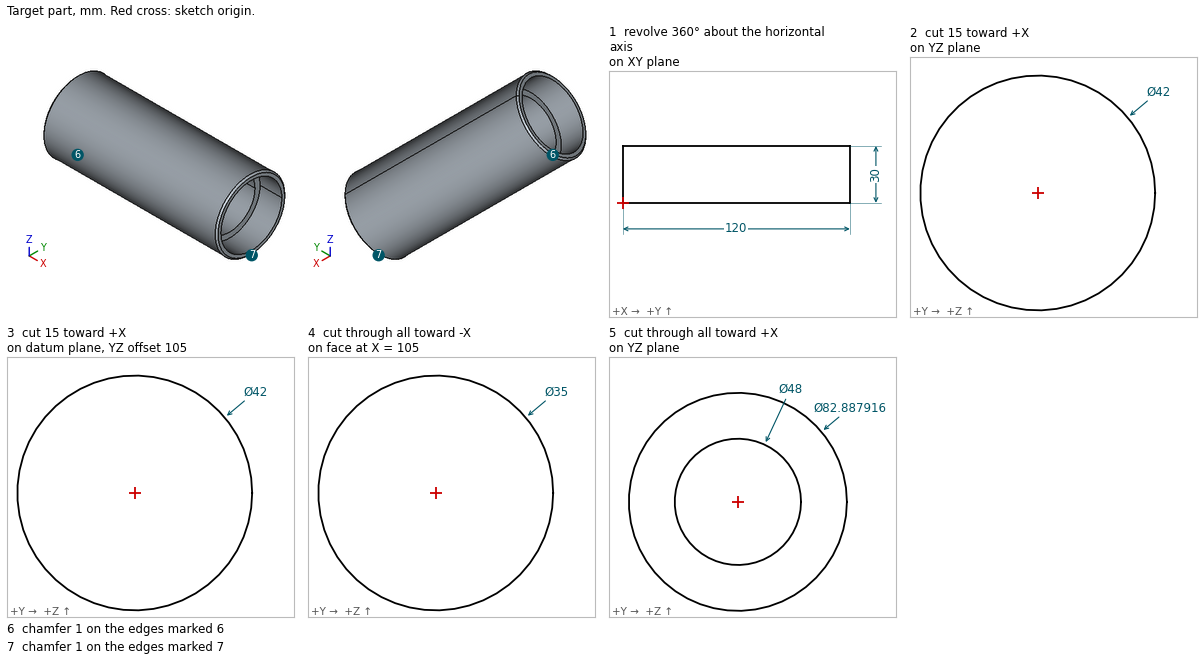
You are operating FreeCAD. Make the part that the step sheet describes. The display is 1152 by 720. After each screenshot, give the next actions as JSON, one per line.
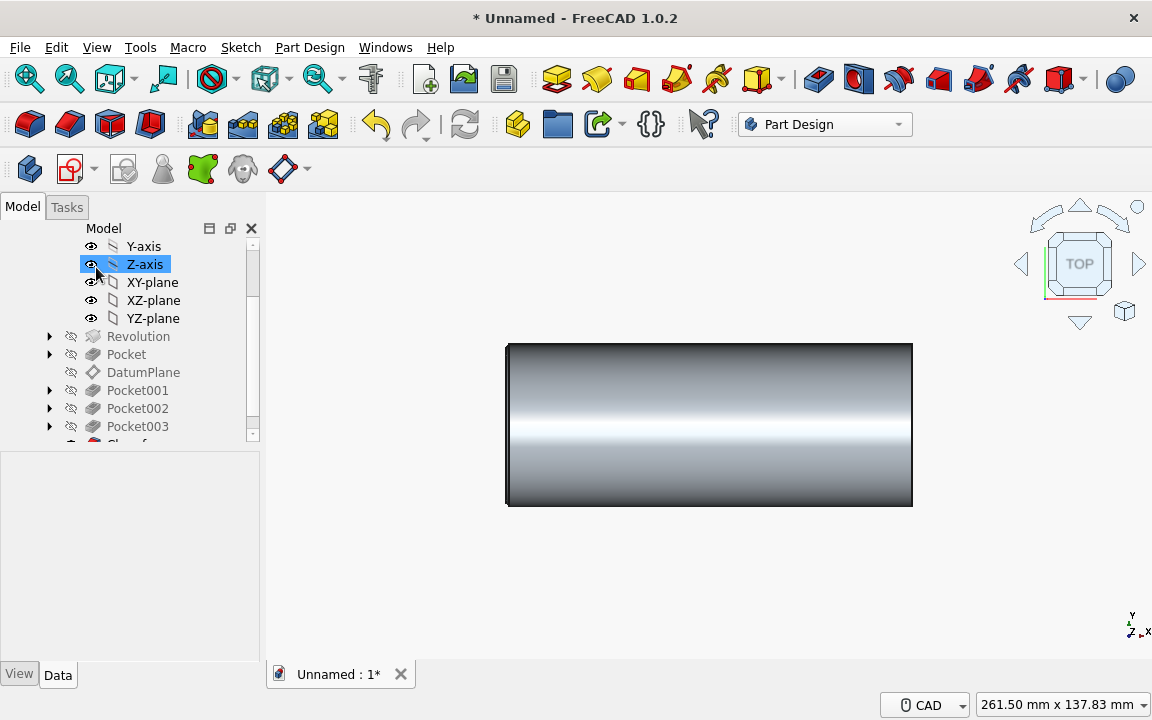
{"action": "left_click", "coordinate": [912, 490]}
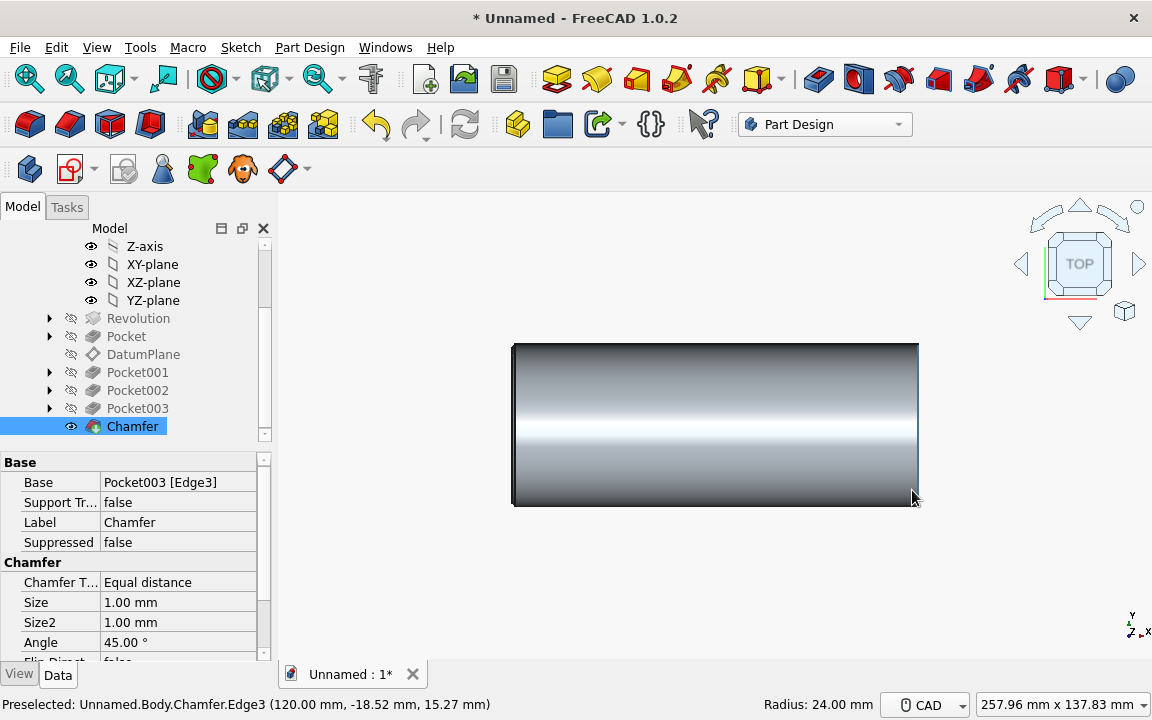
{"action": "left_click", "coordinate": [70, 124]}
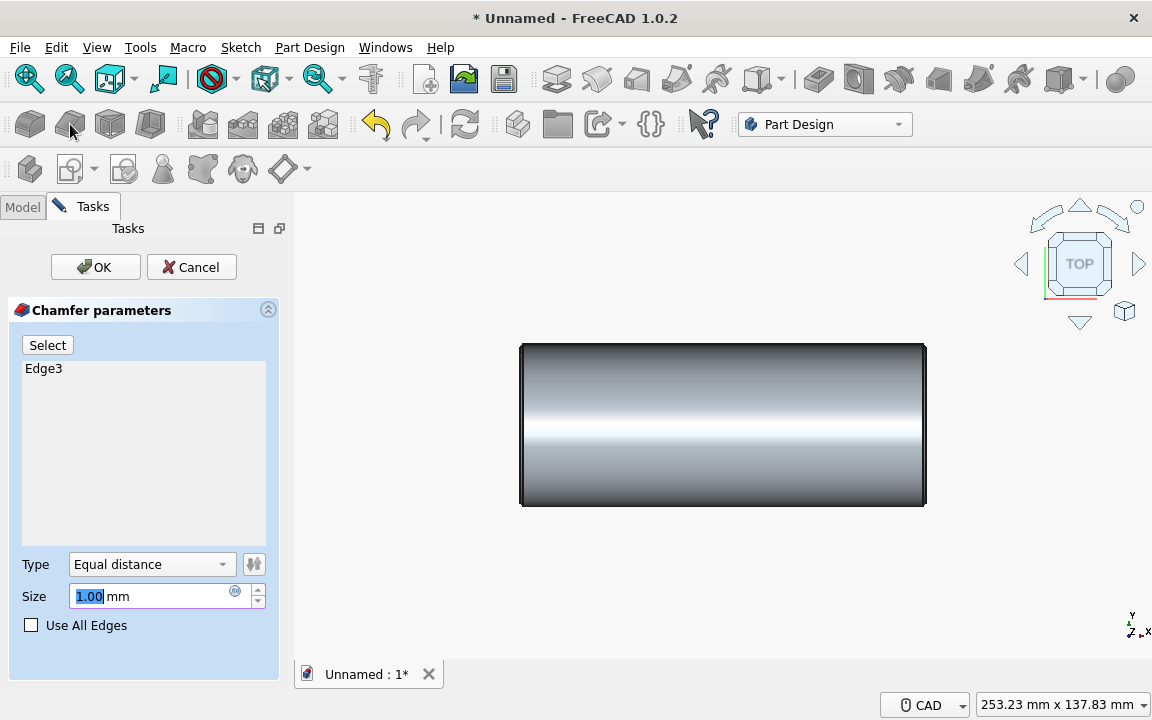
{"action": "type", "text": "1"}
{"action": "key", "text": "Tab"}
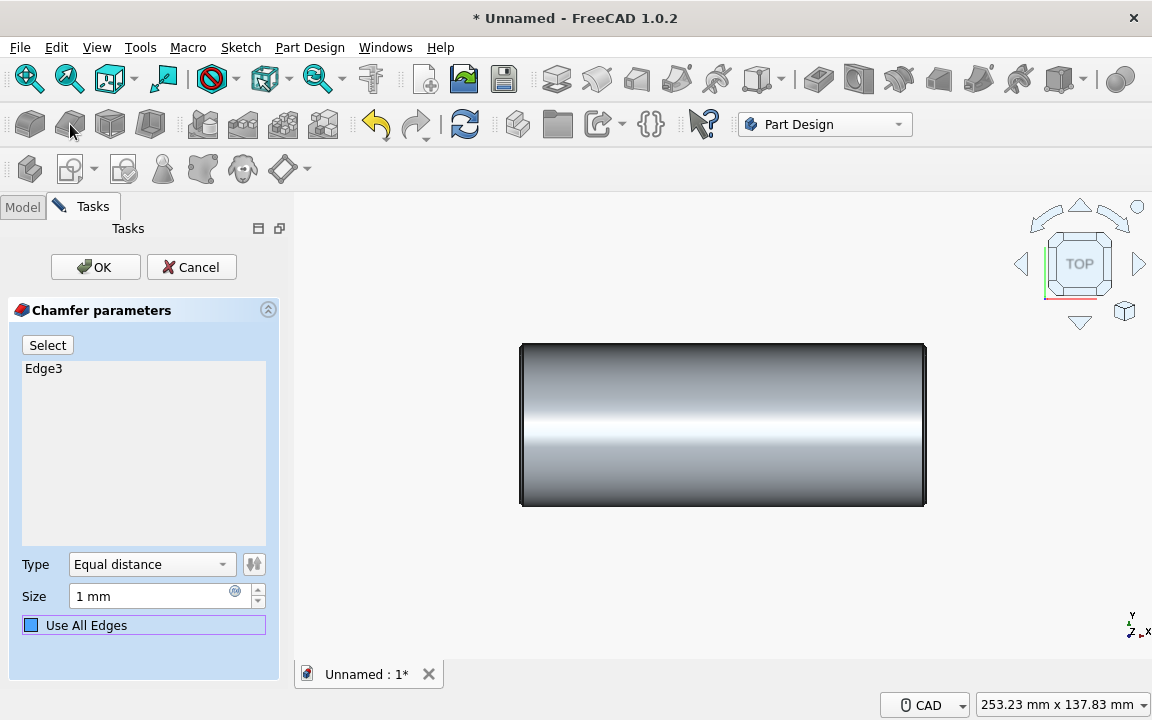
{"action": "left_click", "coordinate": [96, 267]}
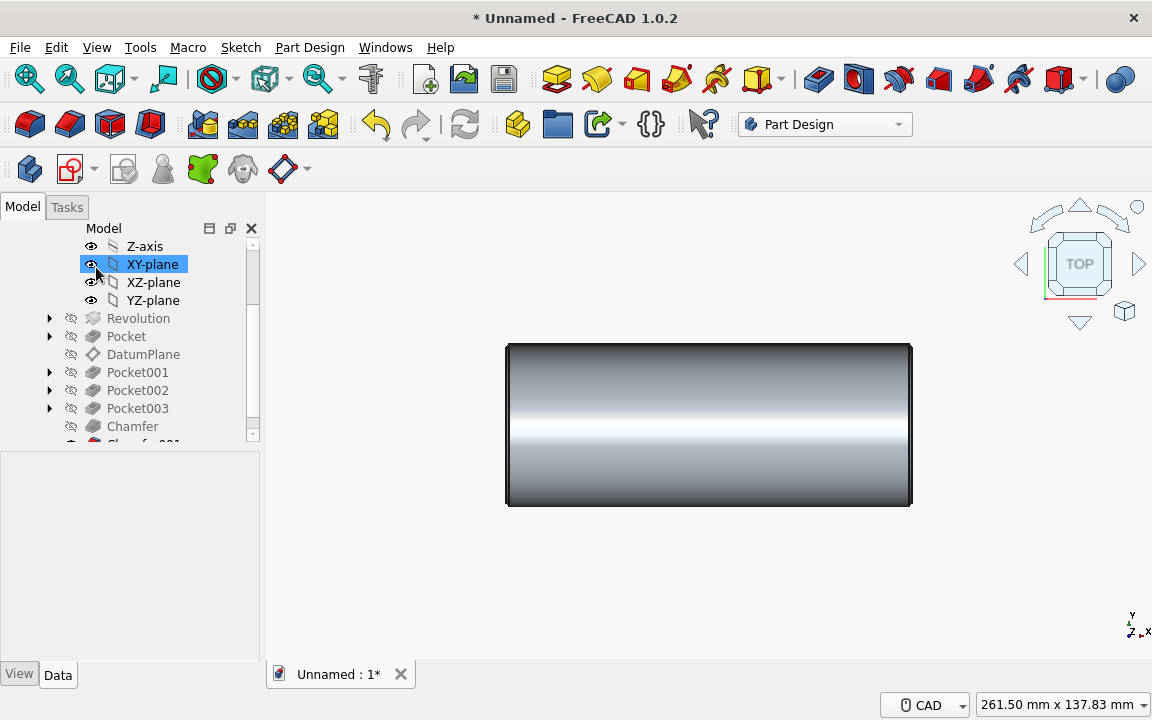
{"action": "key", "text": "0"}